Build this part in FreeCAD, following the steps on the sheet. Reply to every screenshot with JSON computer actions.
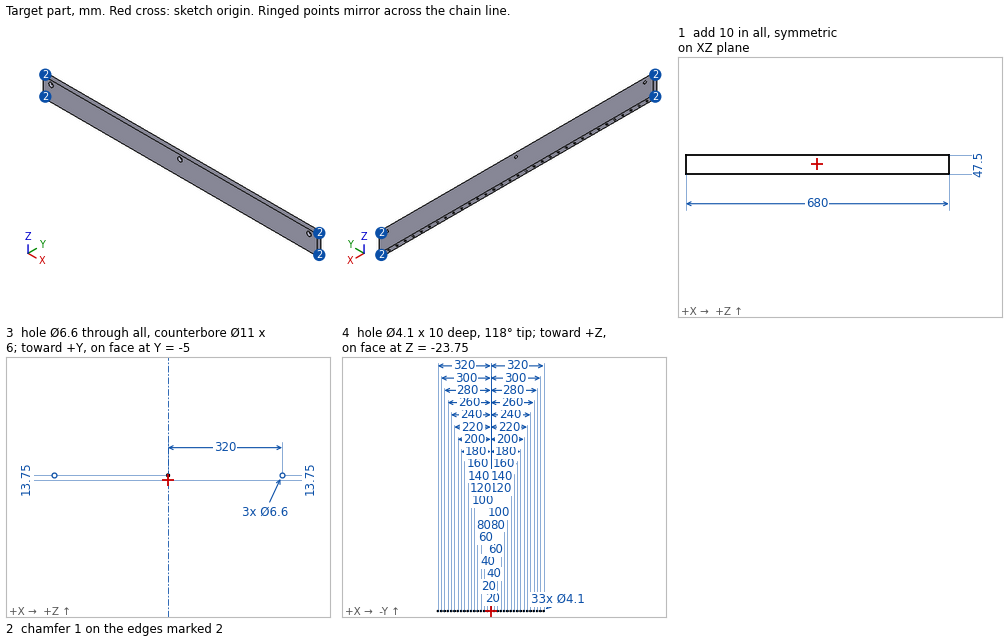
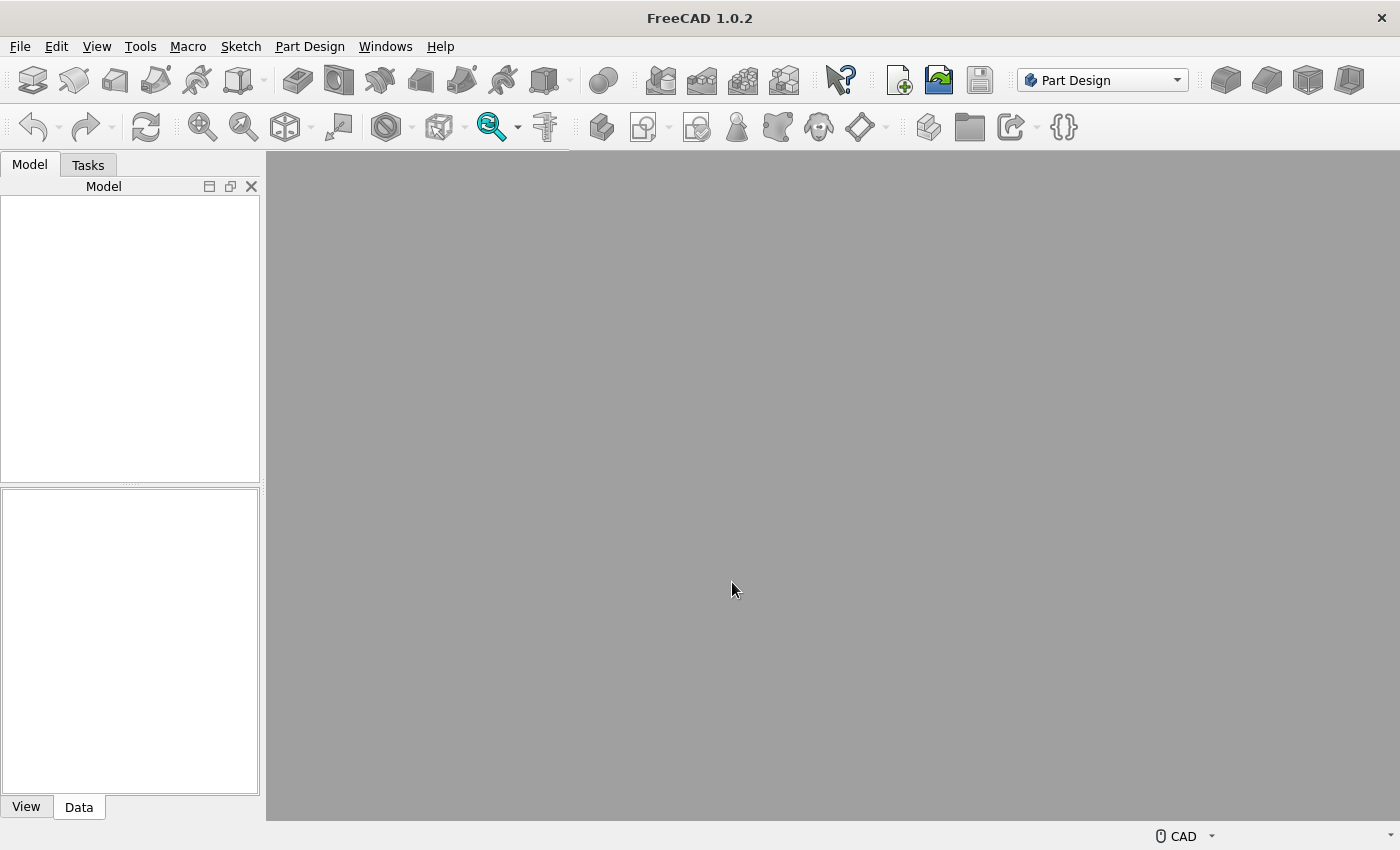
{"action": "left_click", "coordinate": [898, 80]}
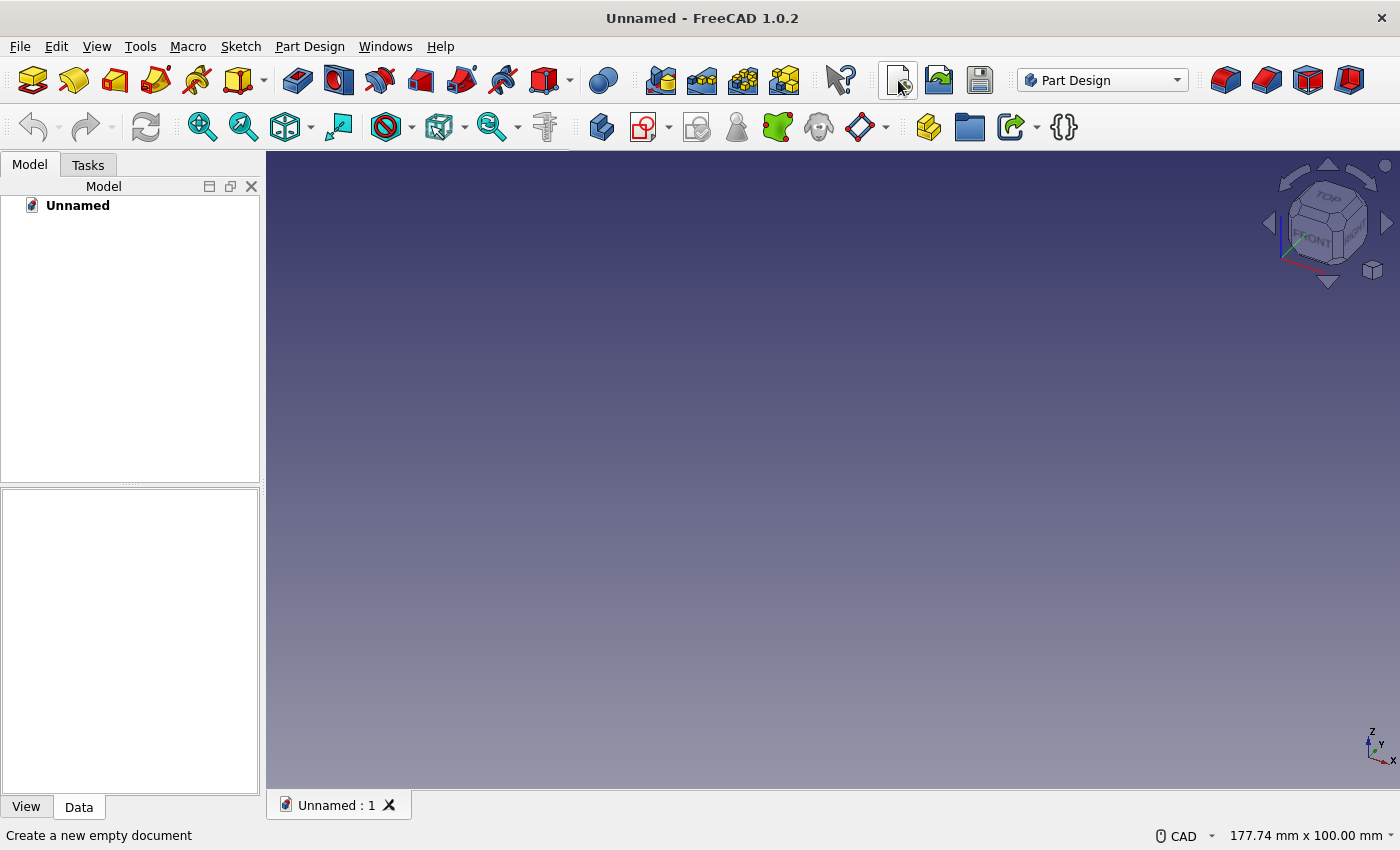
{"action": "left_click", "coordinate": [642, 128]}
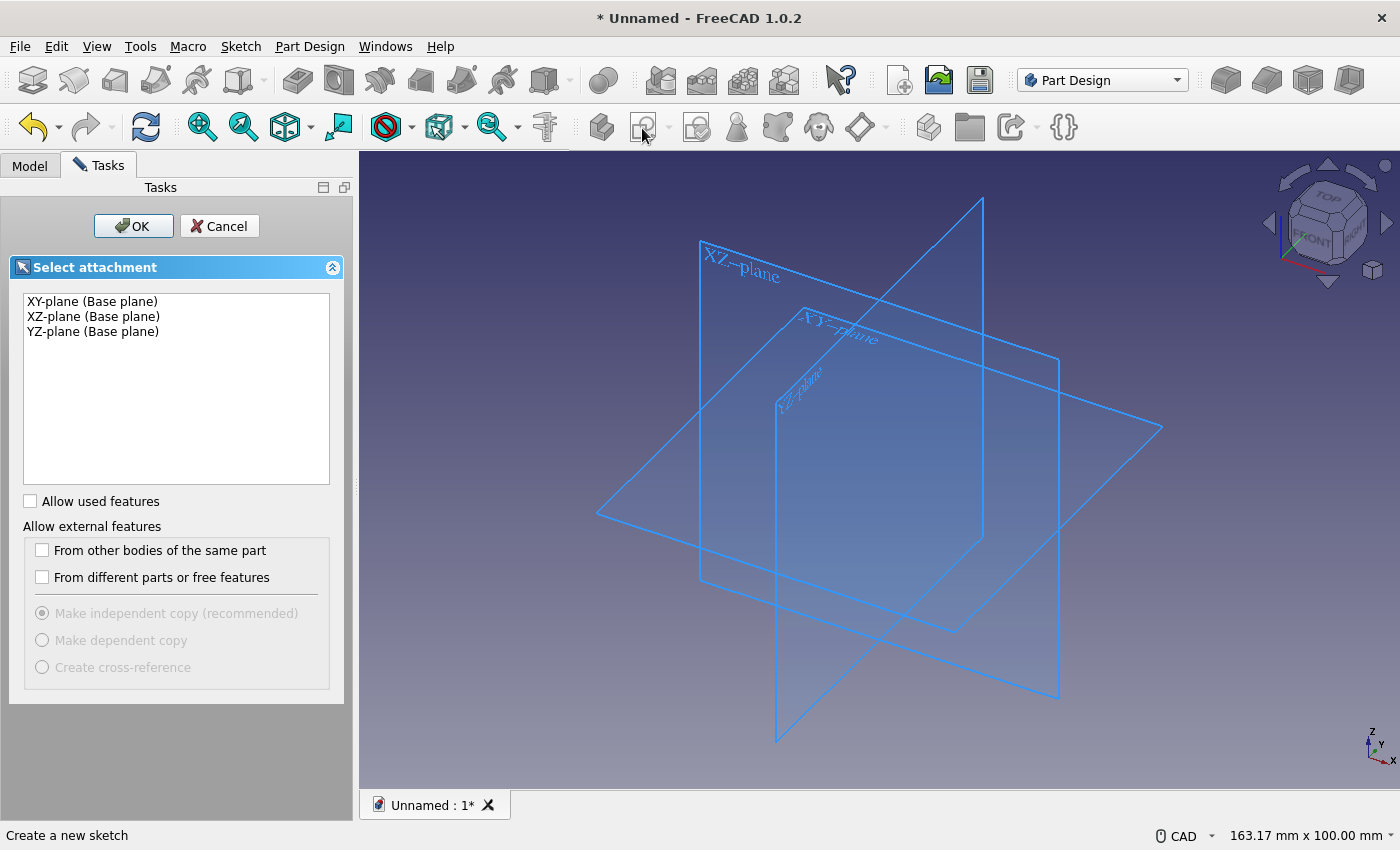
{"action": "left_click", "coordinate": [84, 316]}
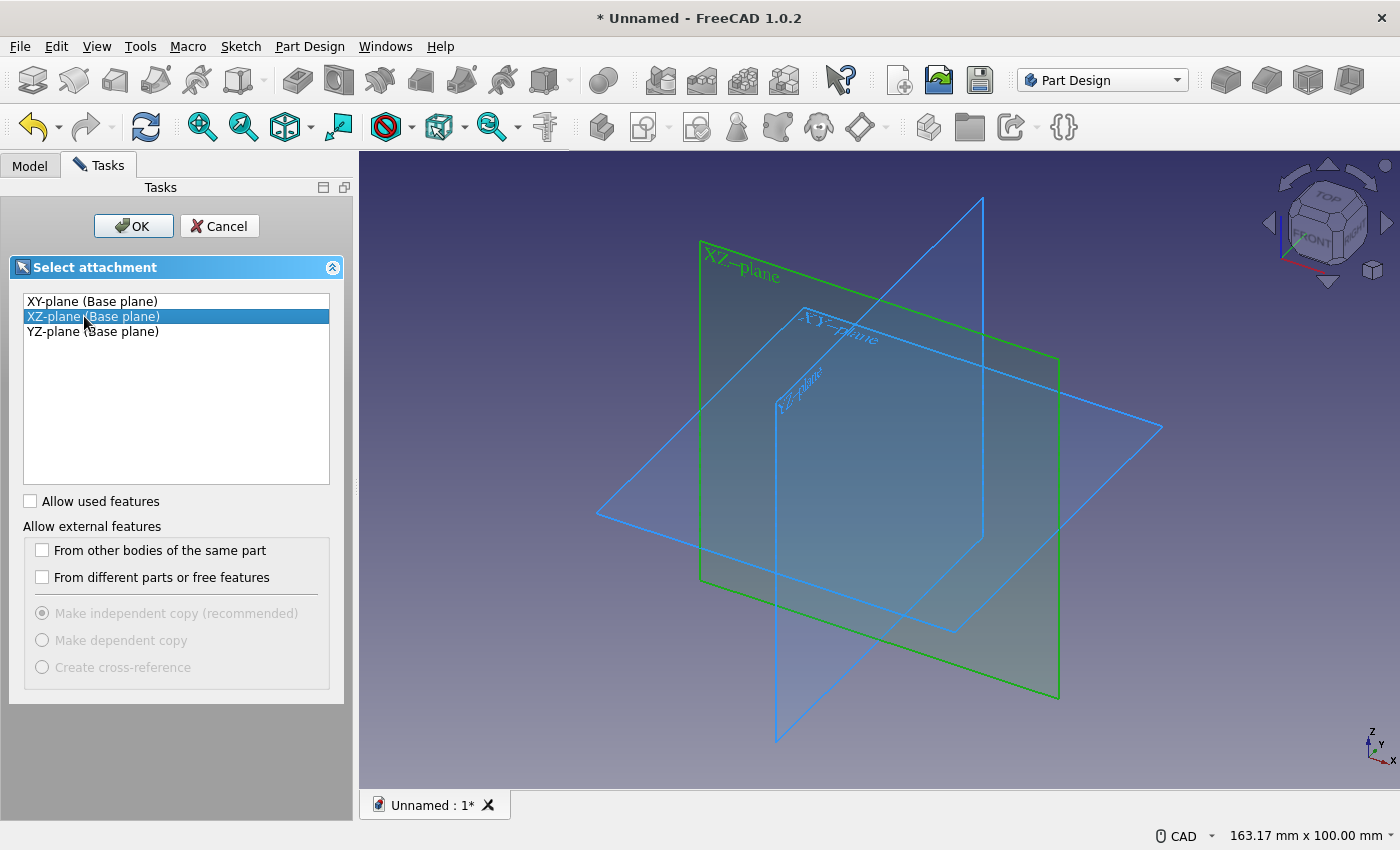
{"action": "left_click", "coordinate": [134, 226]}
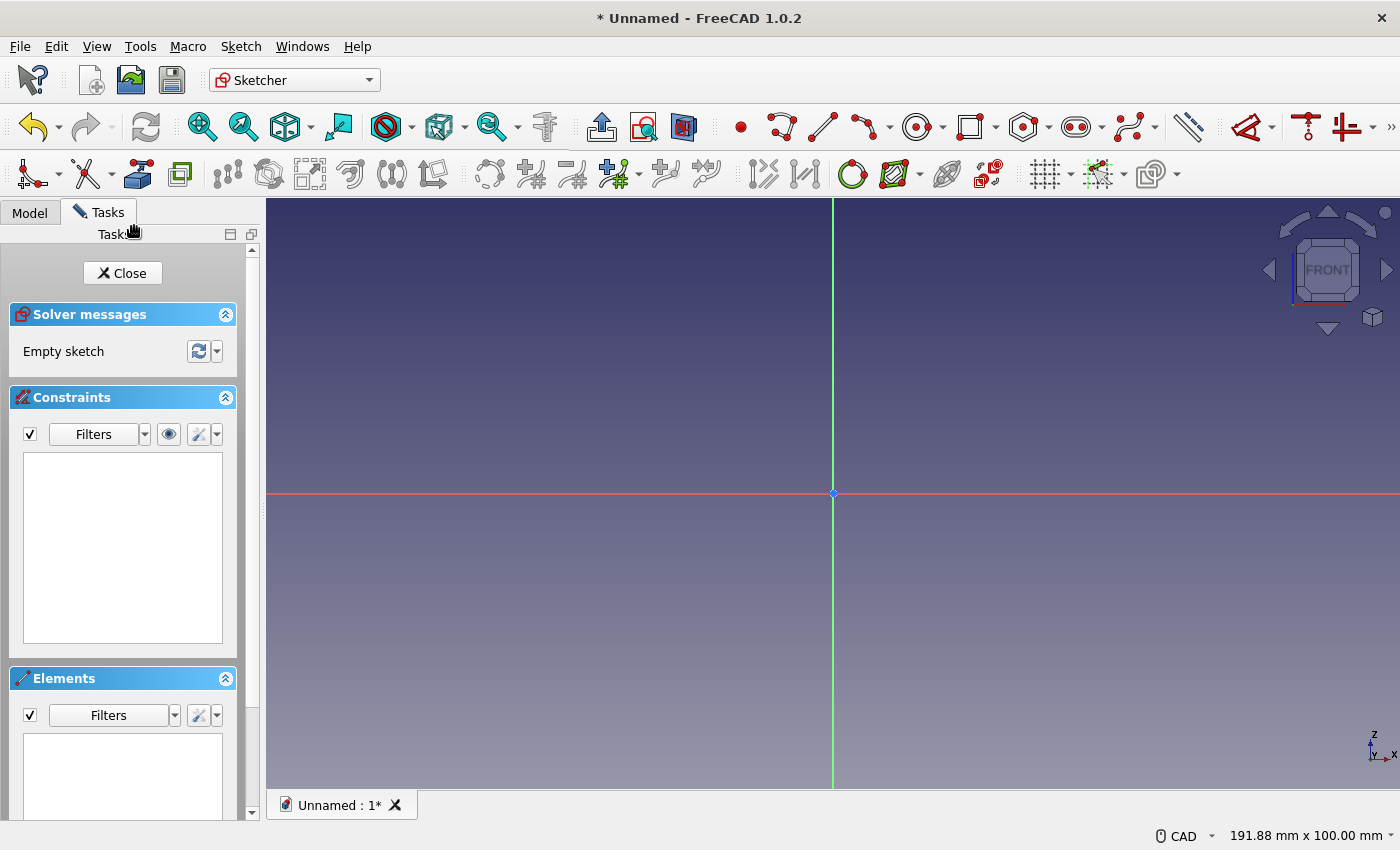
{"action": "scroll", "coordinate": [751, 494], "scroll_direction": "down", "scroll_amount": 9}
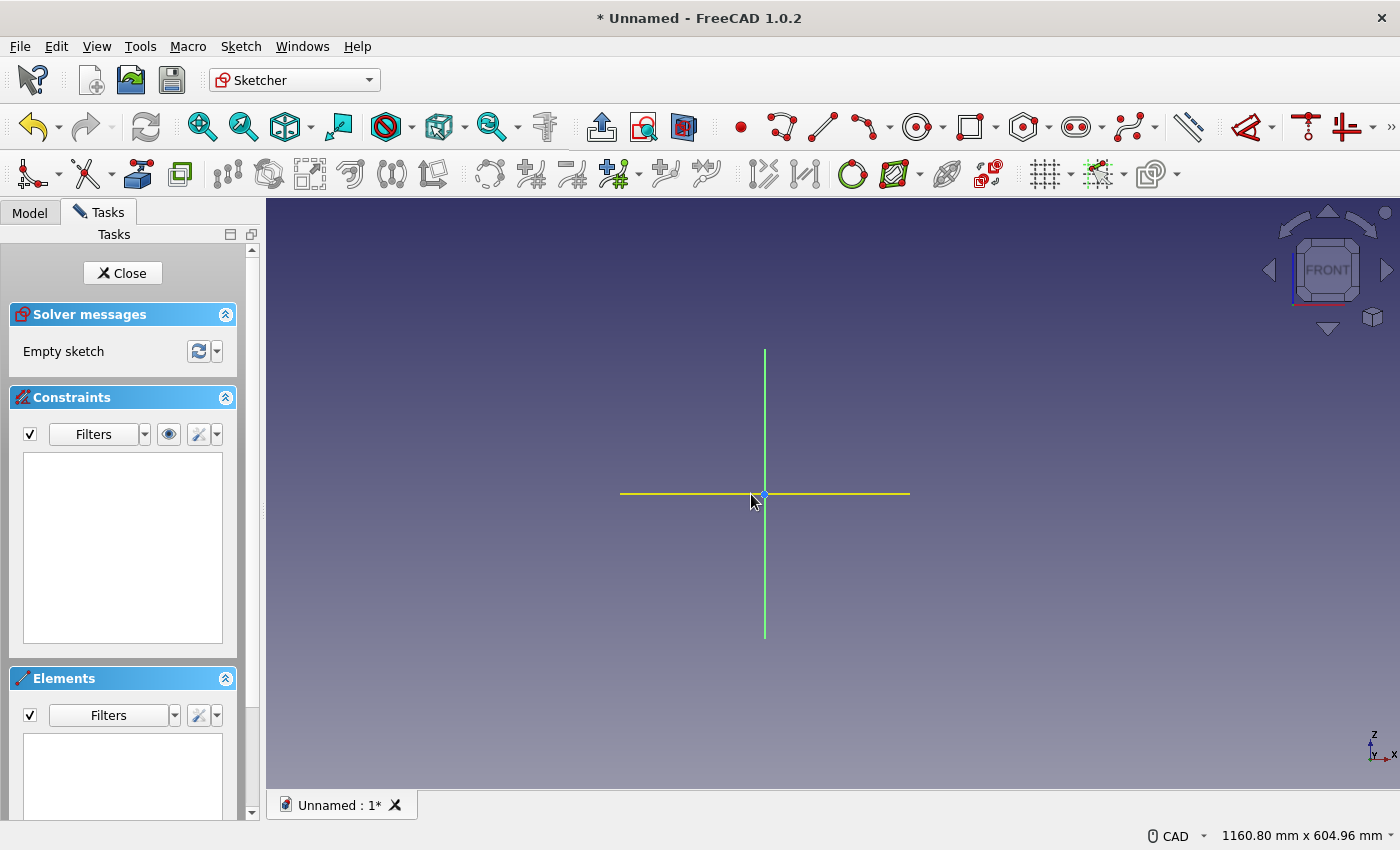
{"action": "left_click", "coordinate": [996, 128]}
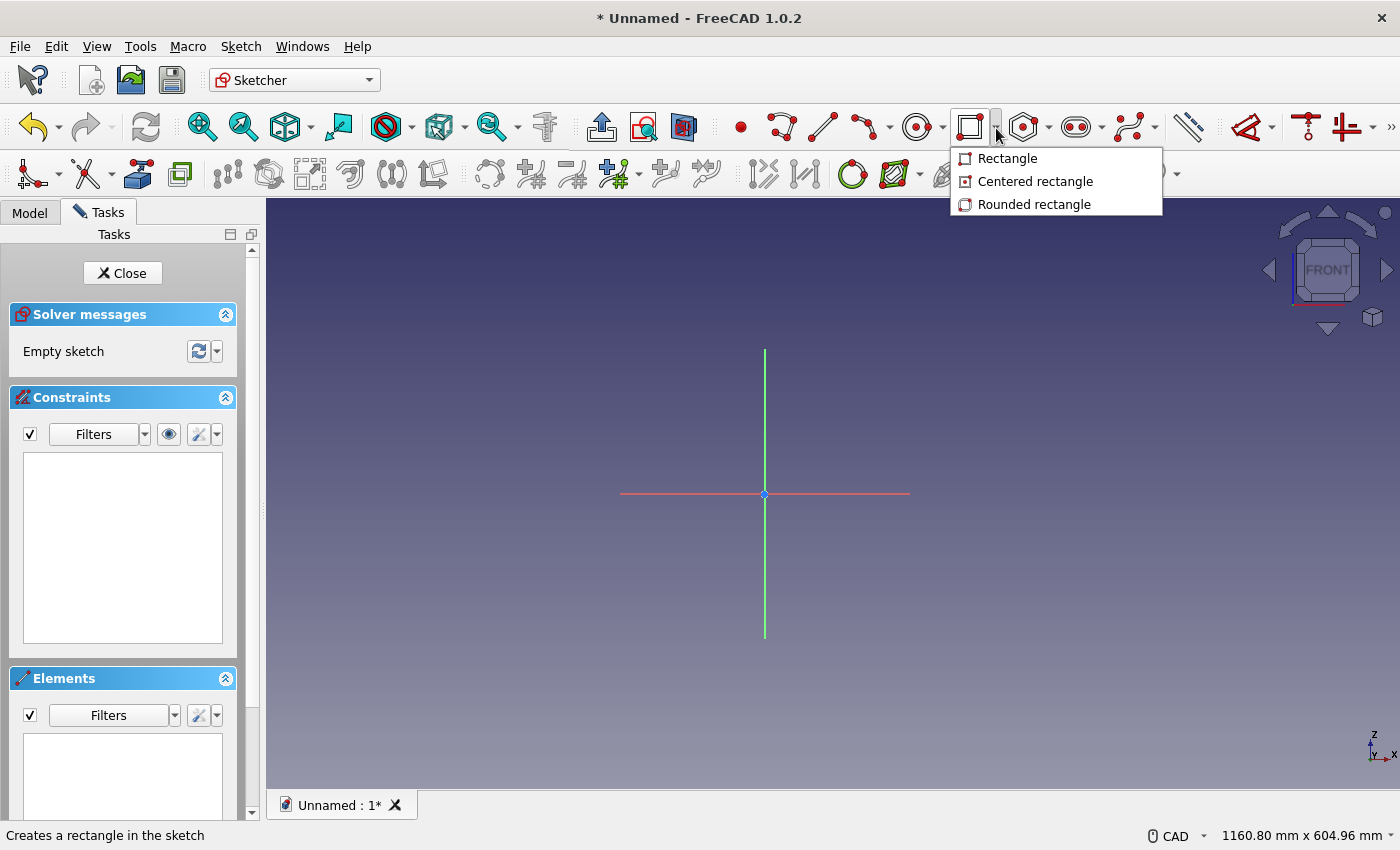
{"action": "left_click", "coordinate": [1056, 182]}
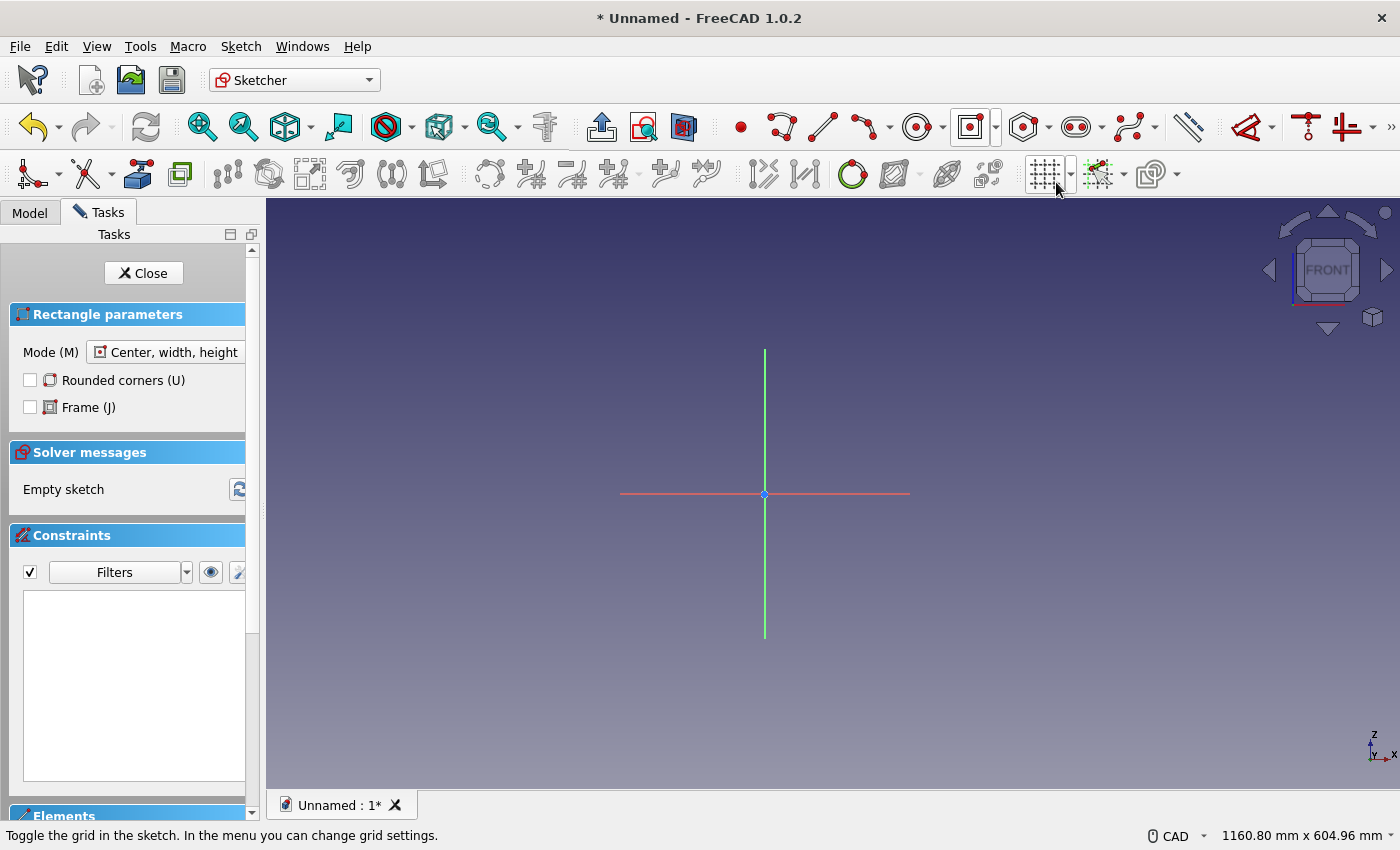
{"action": "left_click", "coordinate": [765, 494]}
{"action": "mouse_move", "coordinate": [1097, 471]}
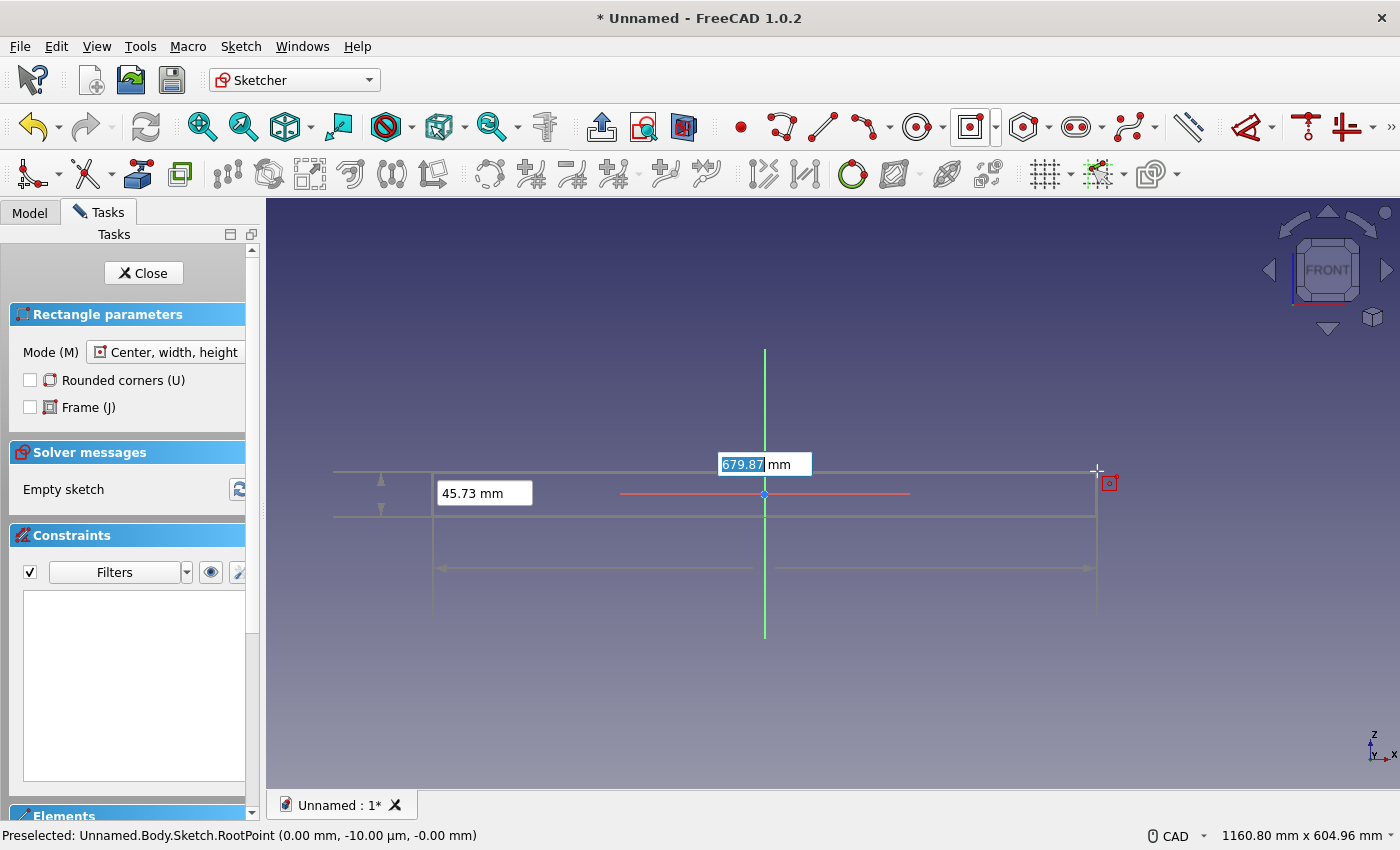
{"action": "type", "text": "680"}
{"action": "key", "text": "Tab"}
{"action": "type", "text": "47.5"}
{"action": "key", "text": "Return"}
{"action": "key", "text": "Escape"}